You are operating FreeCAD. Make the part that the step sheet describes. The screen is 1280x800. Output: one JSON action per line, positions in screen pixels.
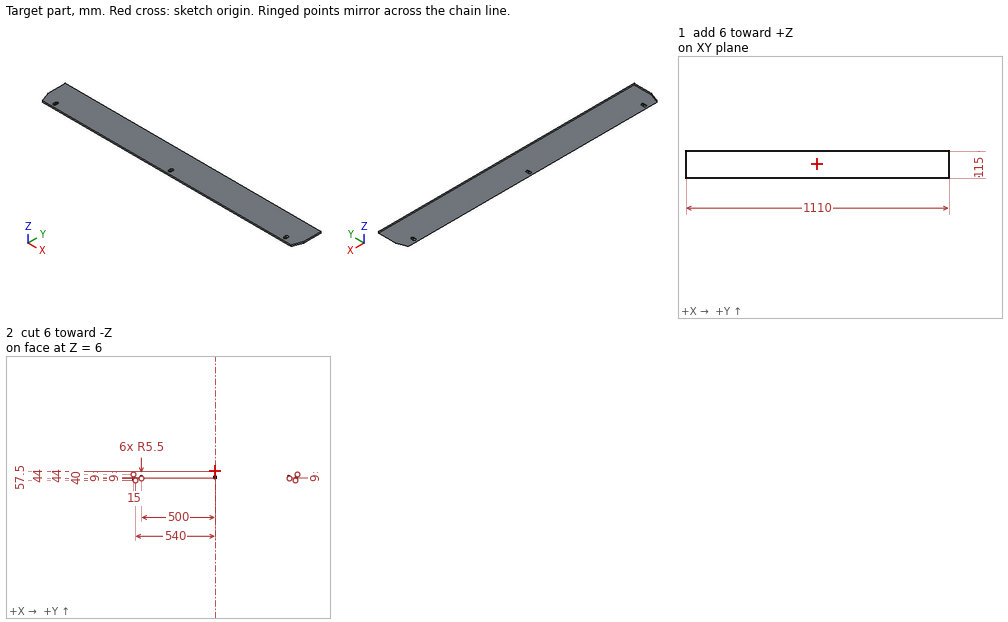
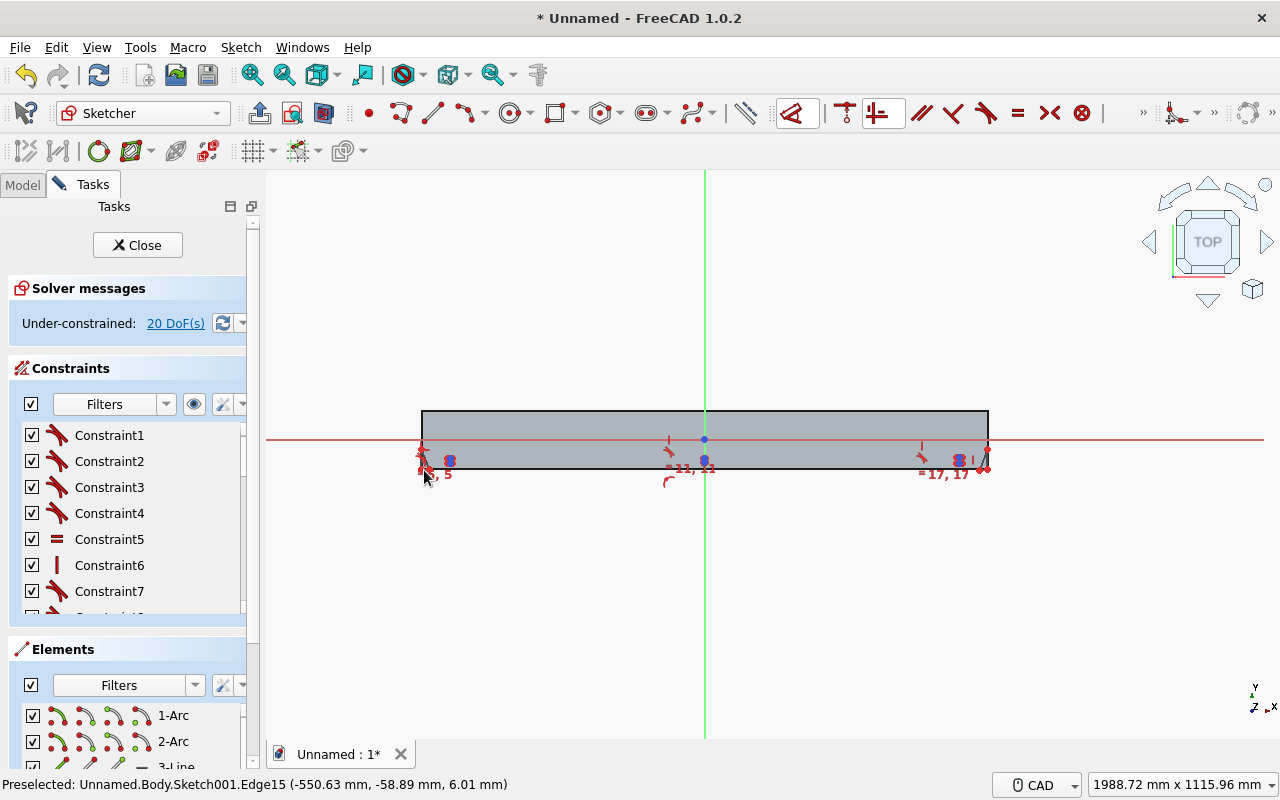
{"action": "scroll", "coordinate": [982, 470], "scroll_direction": "up", "scroll_amount": 10}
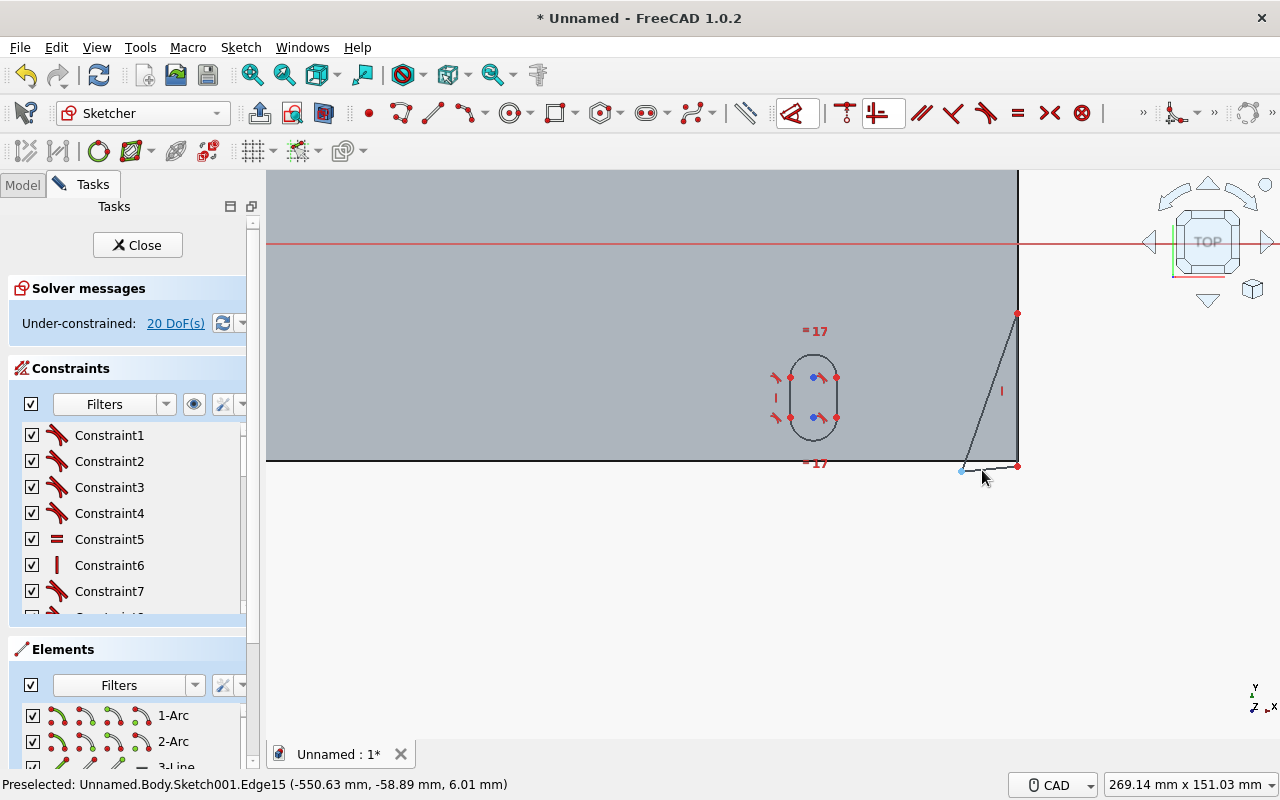
{"action": "left_click", "coordinate": [978, 470]}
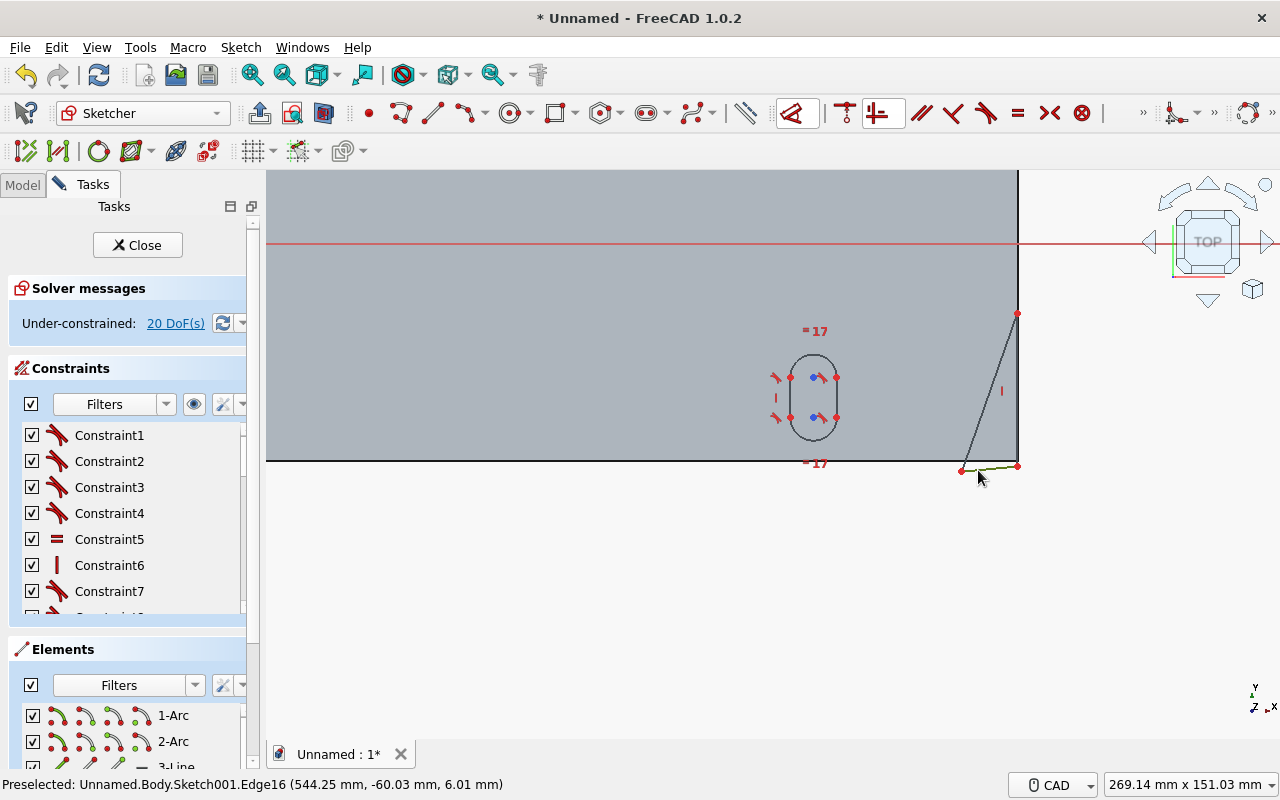
{"action": "left_click", "coordinate": [900, 114]}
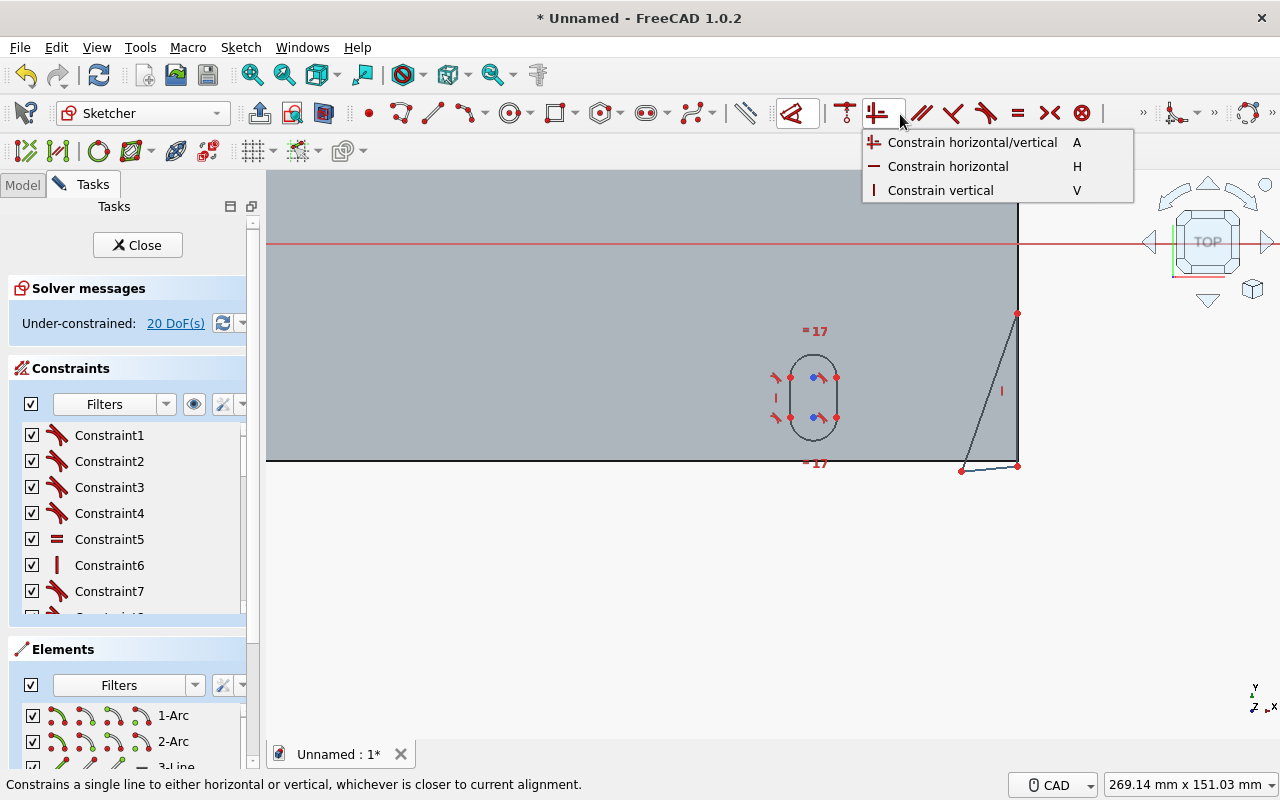
{"action": "left_click", "coordinate": [998, 166]}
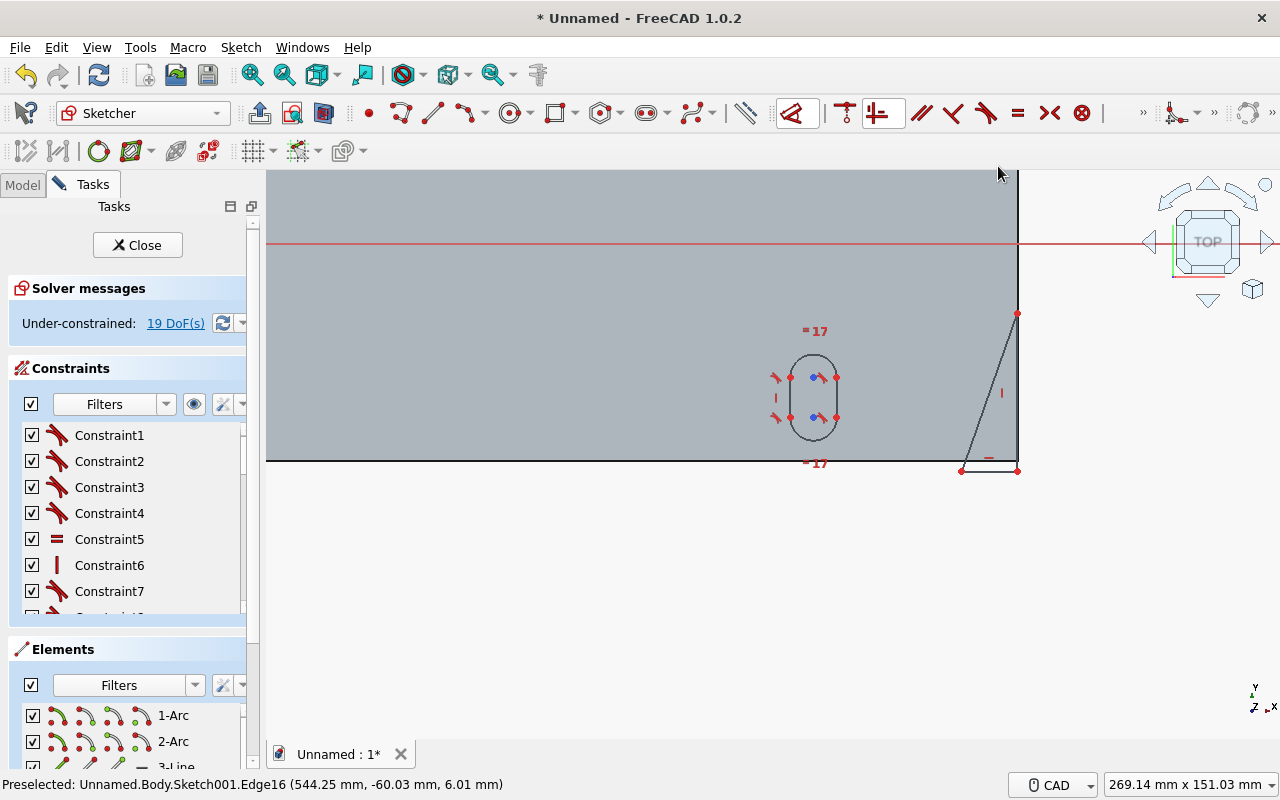
{"action": "scroll", "coordinate": [983, 470], "scroll_direction": "down", "scroll_amount": 10}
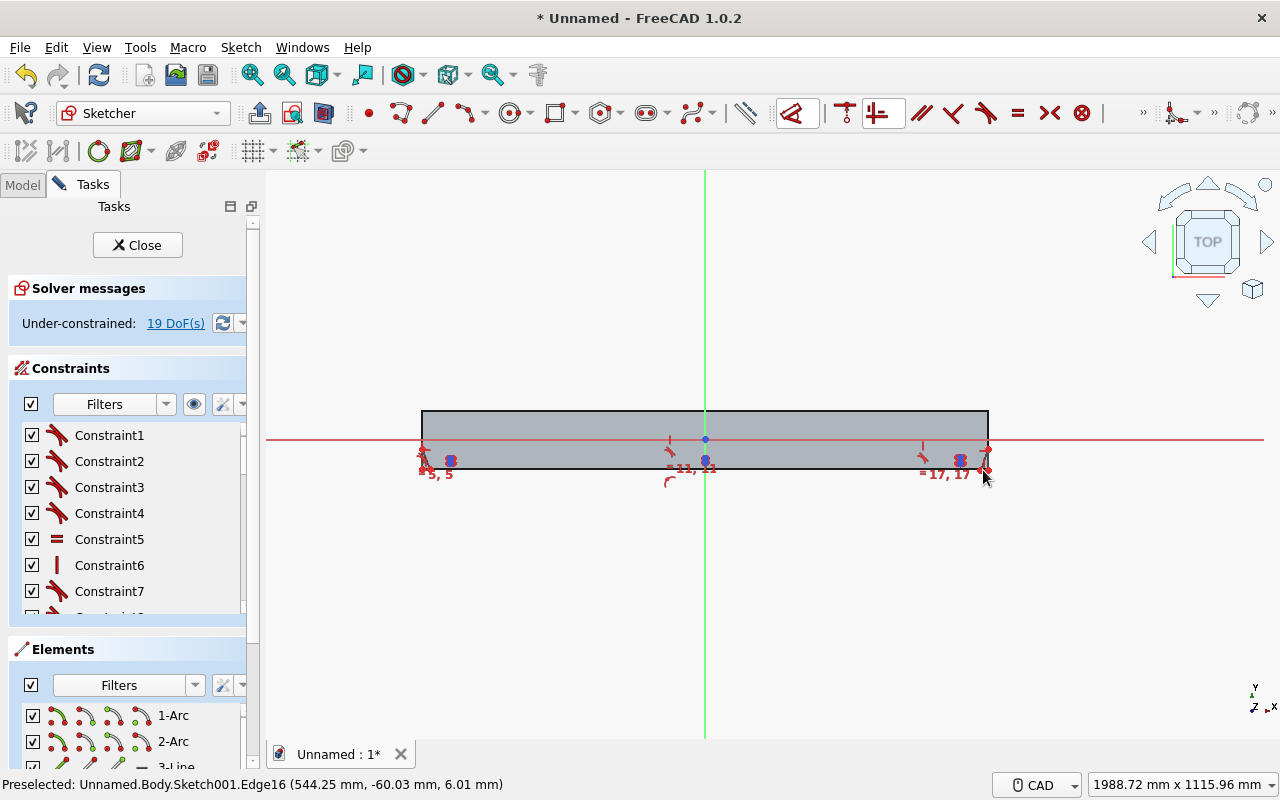
{"action": "scroll", "coordinate": [449, 466], "scroll_direction": "up", "scroll_amount": 10}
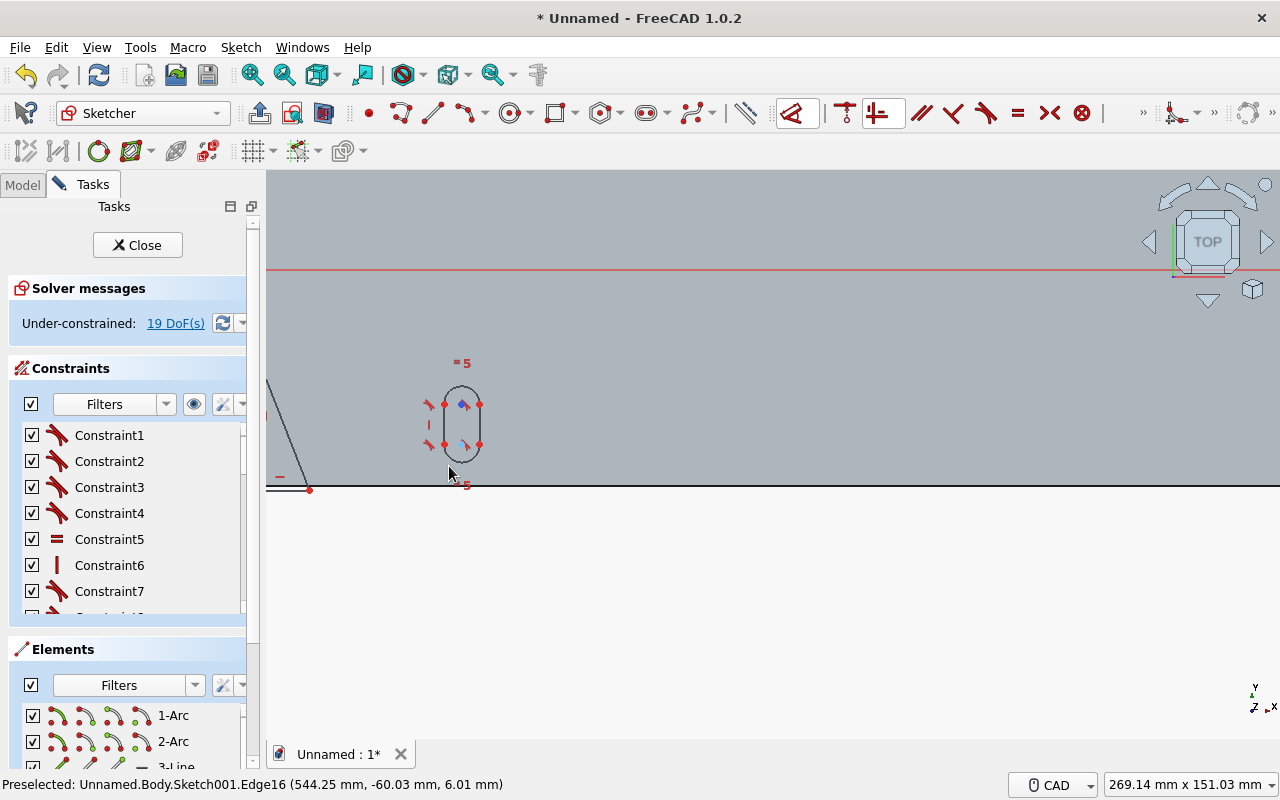
{"action": "left_click", "coordinate": [451, 459]}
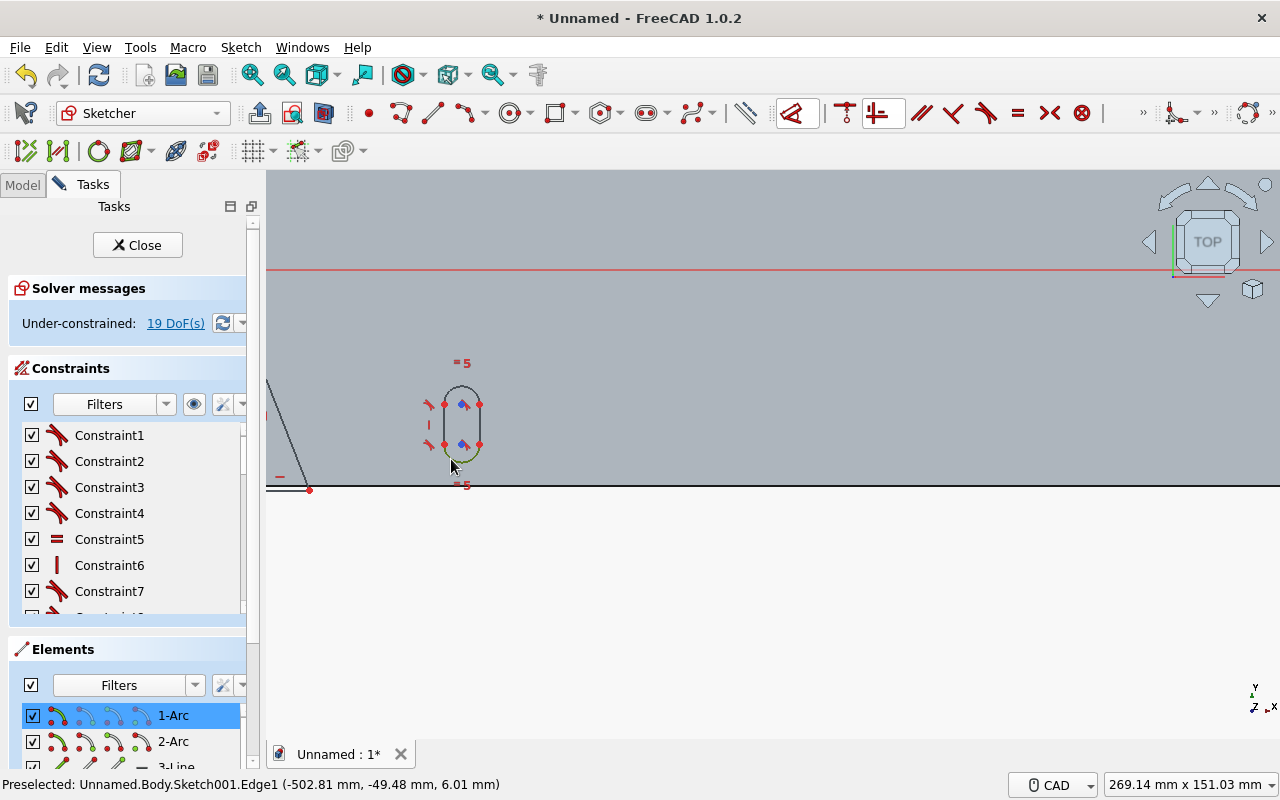
{"action": "scroll", "coordinate": [448, 466], "scroll_direction": "down", "scroll_amount": 10}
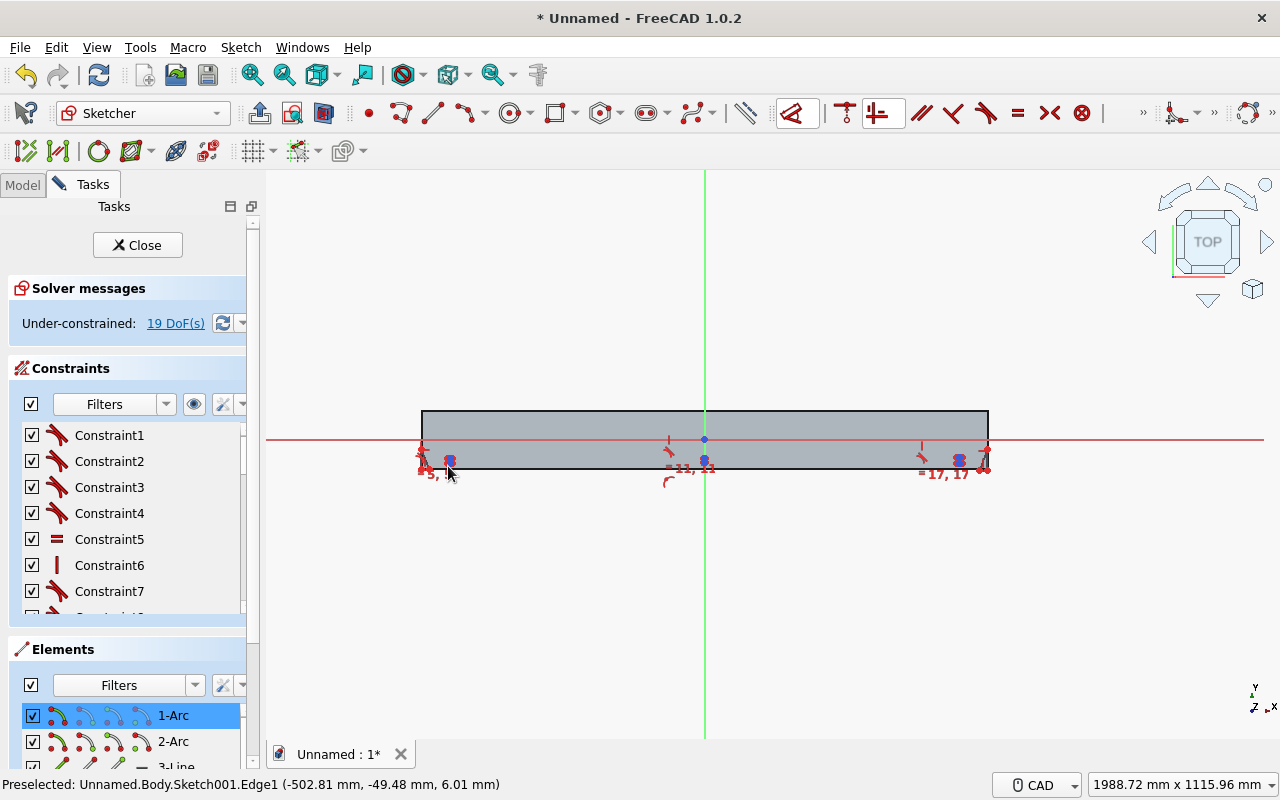
{"action": "scroll", "coordinate": [705, 464], "scroll_direction": "up", "scroll_amount": 14}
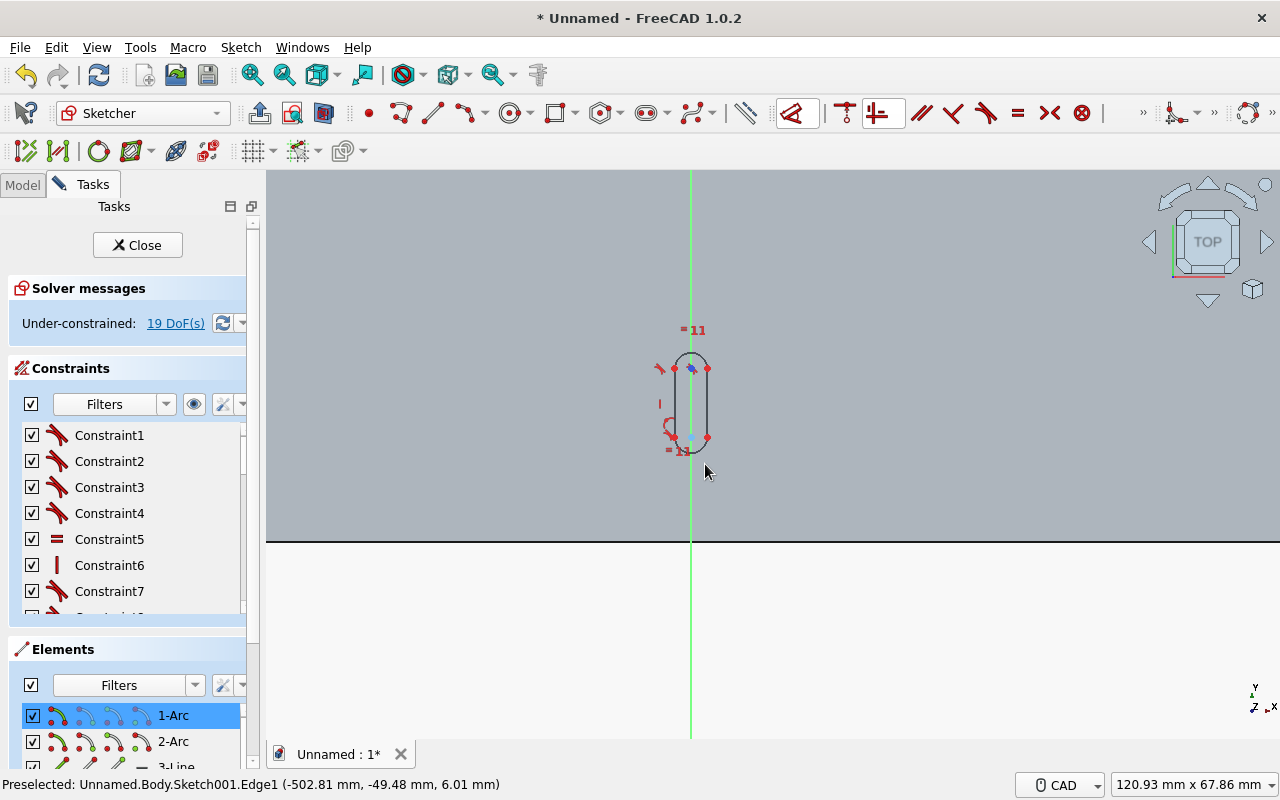
{"action": "left_click", "coordinate": [691, 453]}